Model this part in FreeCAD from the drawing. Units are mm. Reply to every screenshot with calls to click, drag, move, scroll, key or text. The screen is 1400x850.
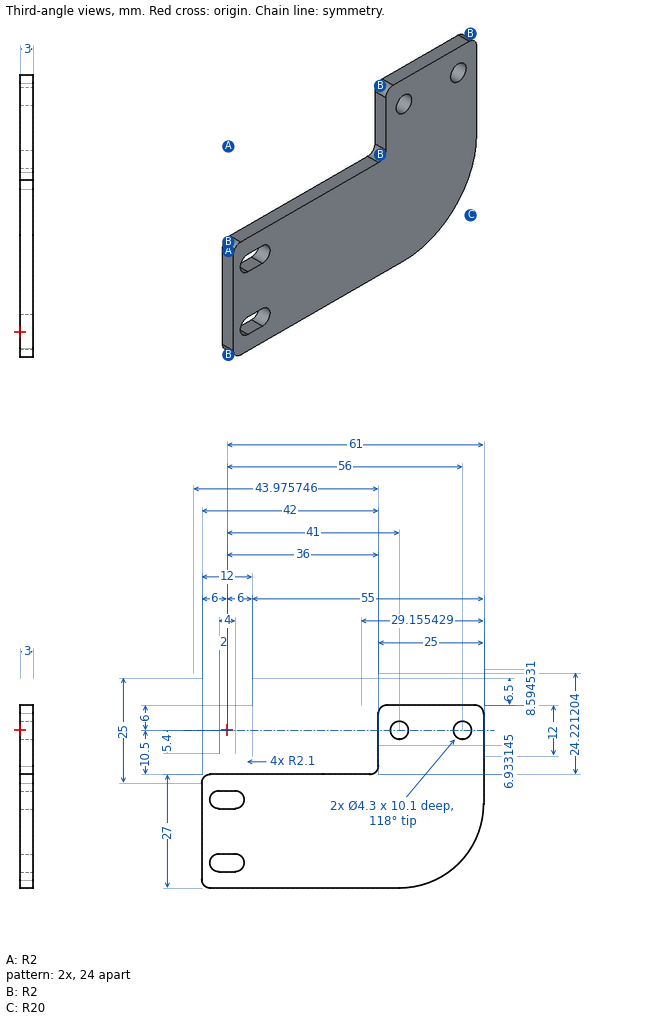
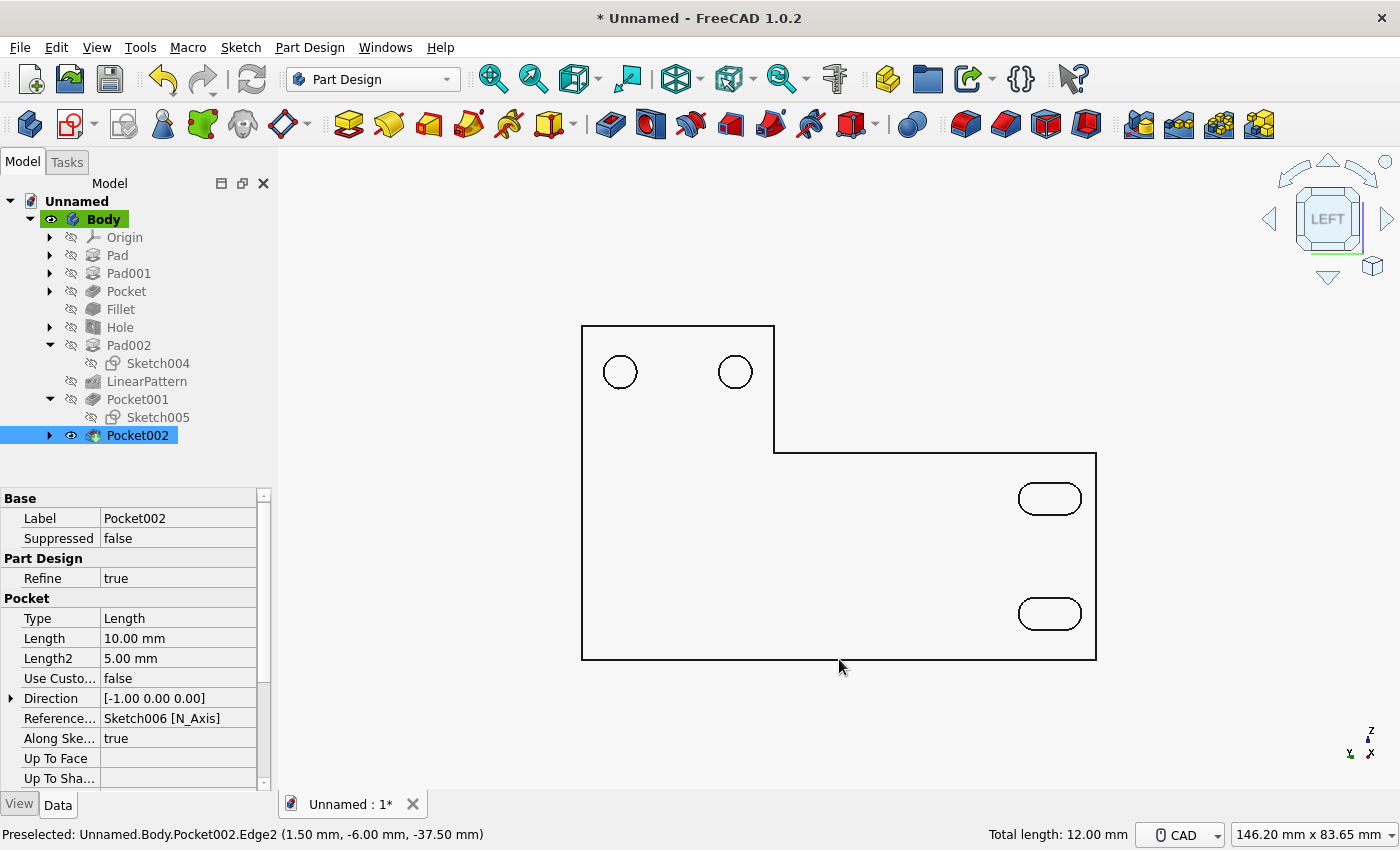
key(0)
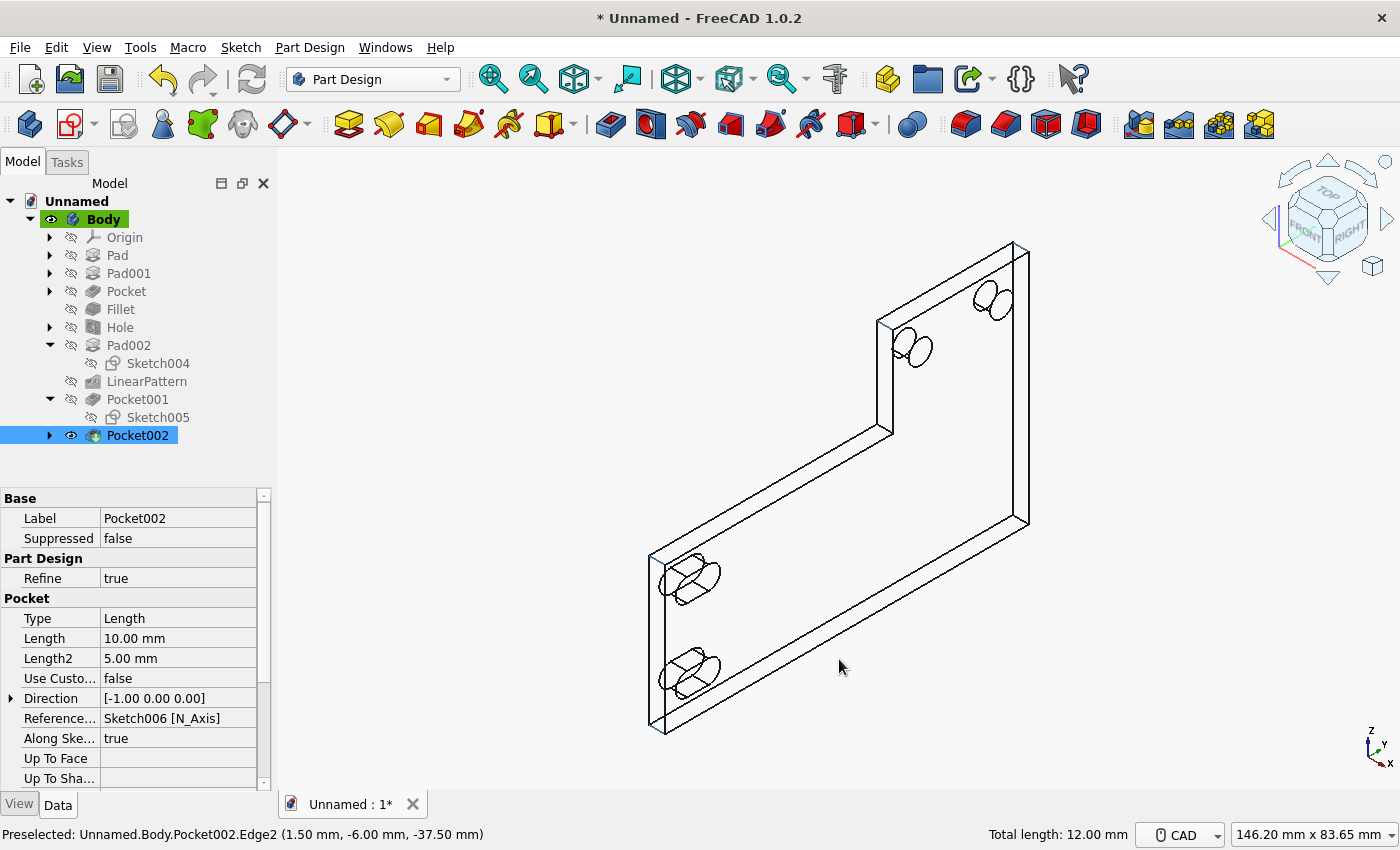
click(885, 428, ctrl)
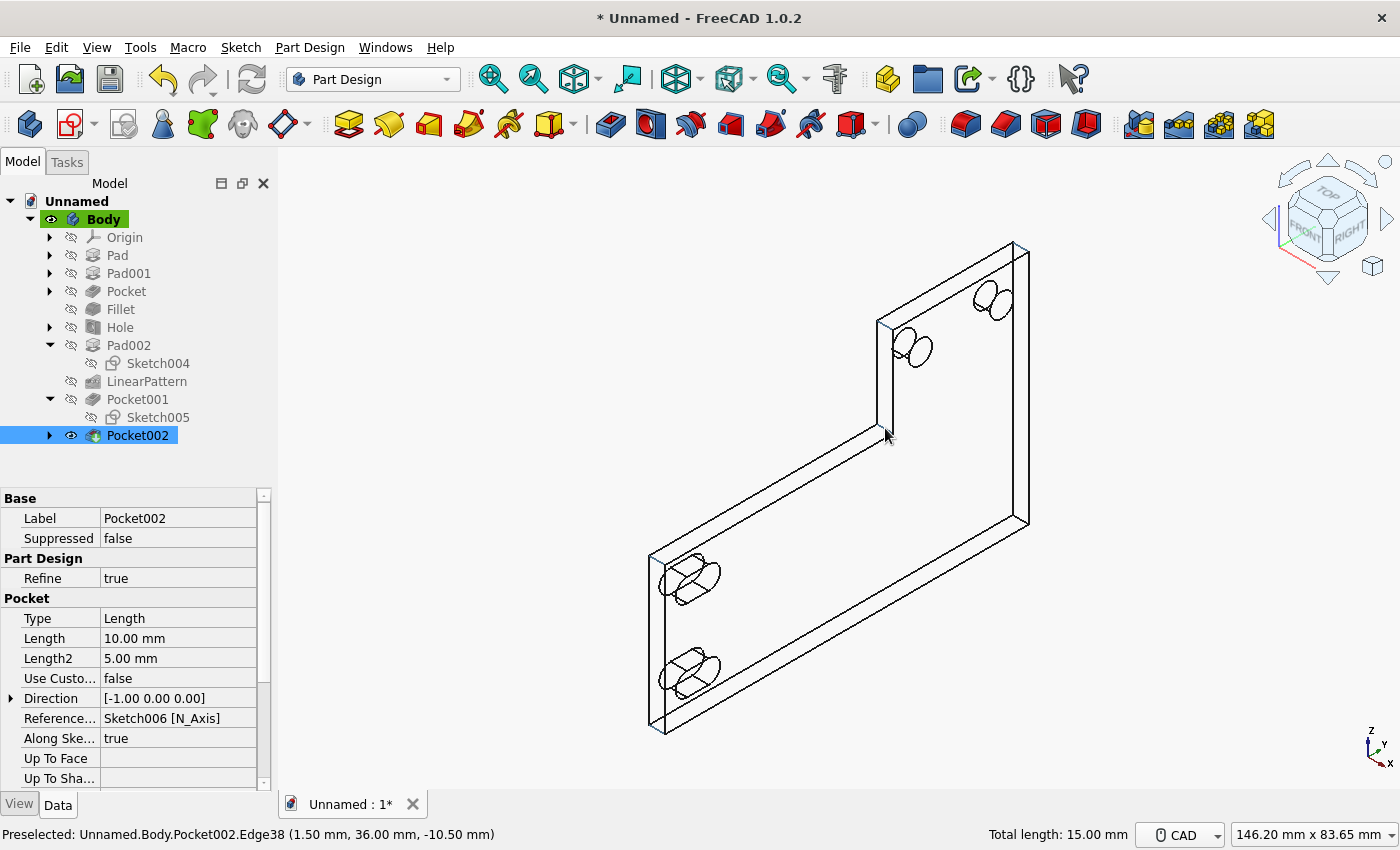
key(v)
key(1)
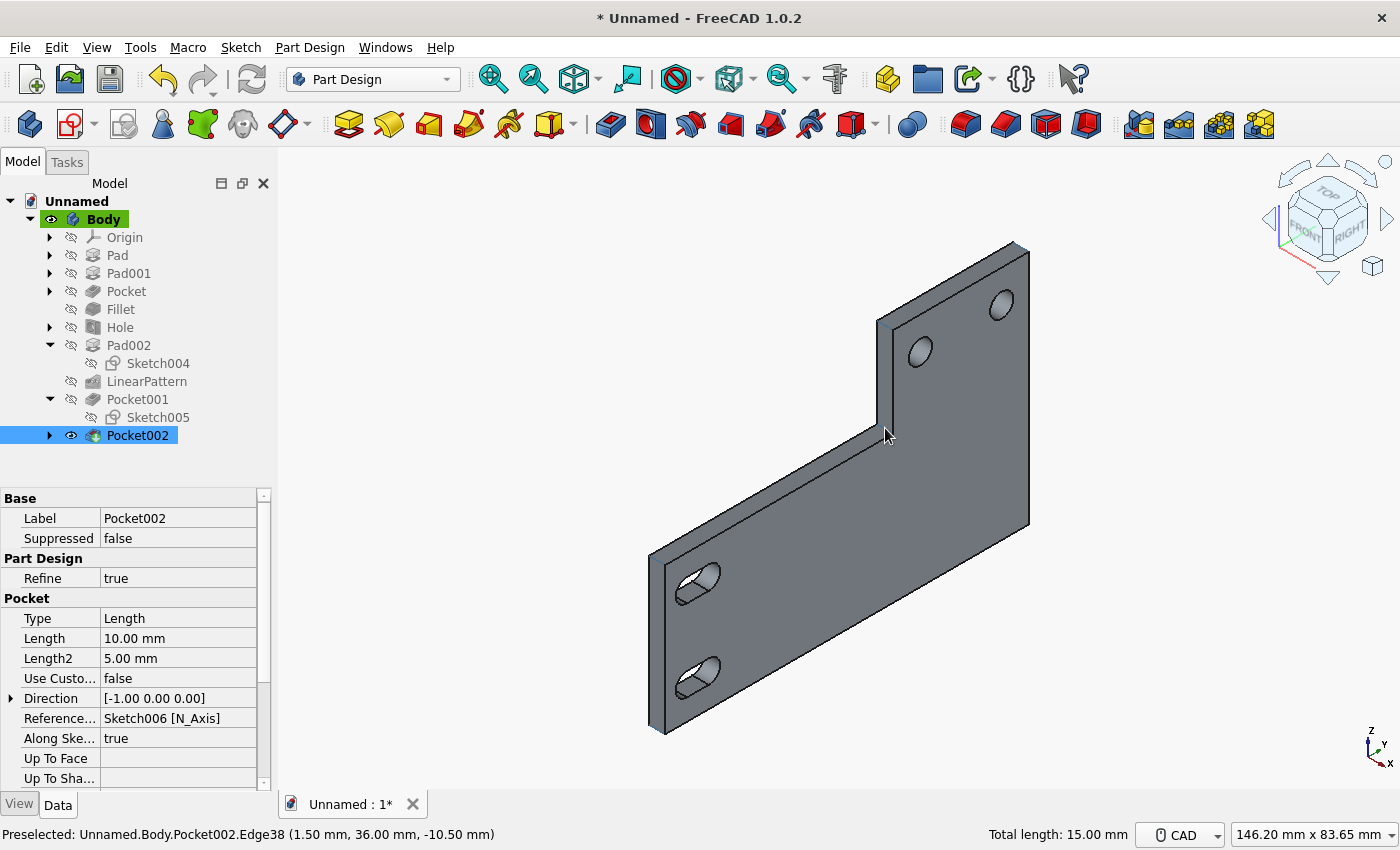
click(966, 124)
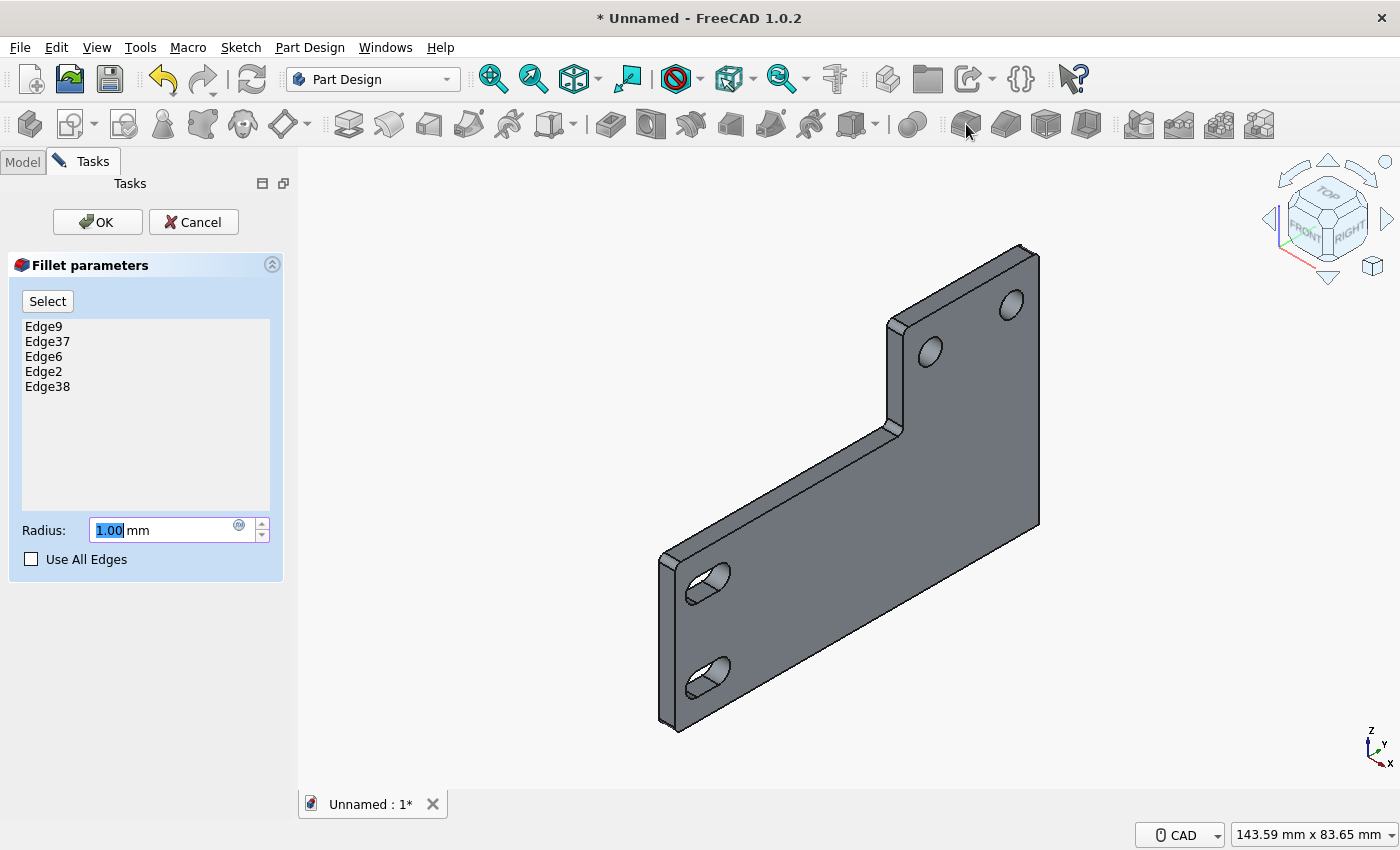
text(2)
key(Tab)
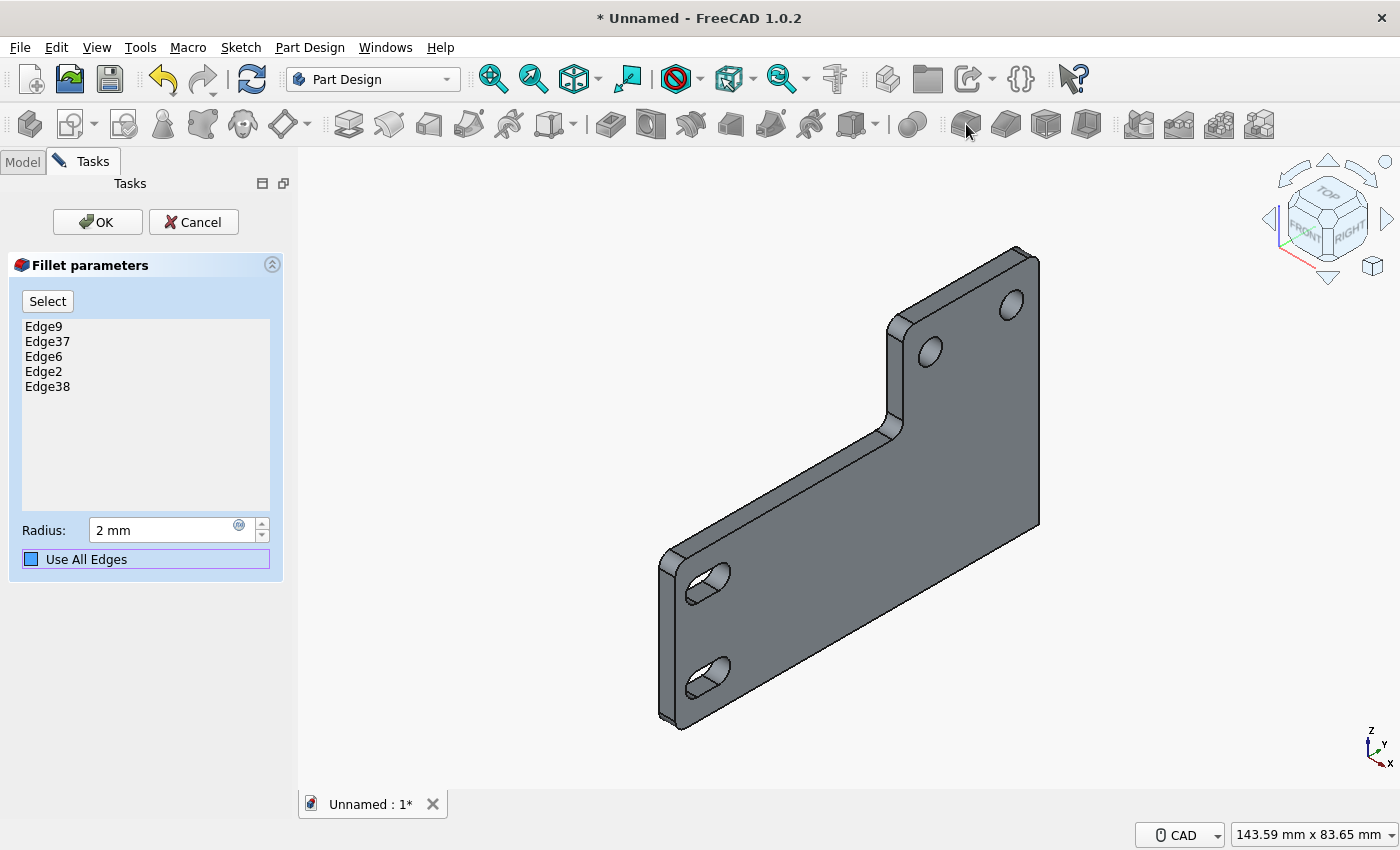
click(98, 222)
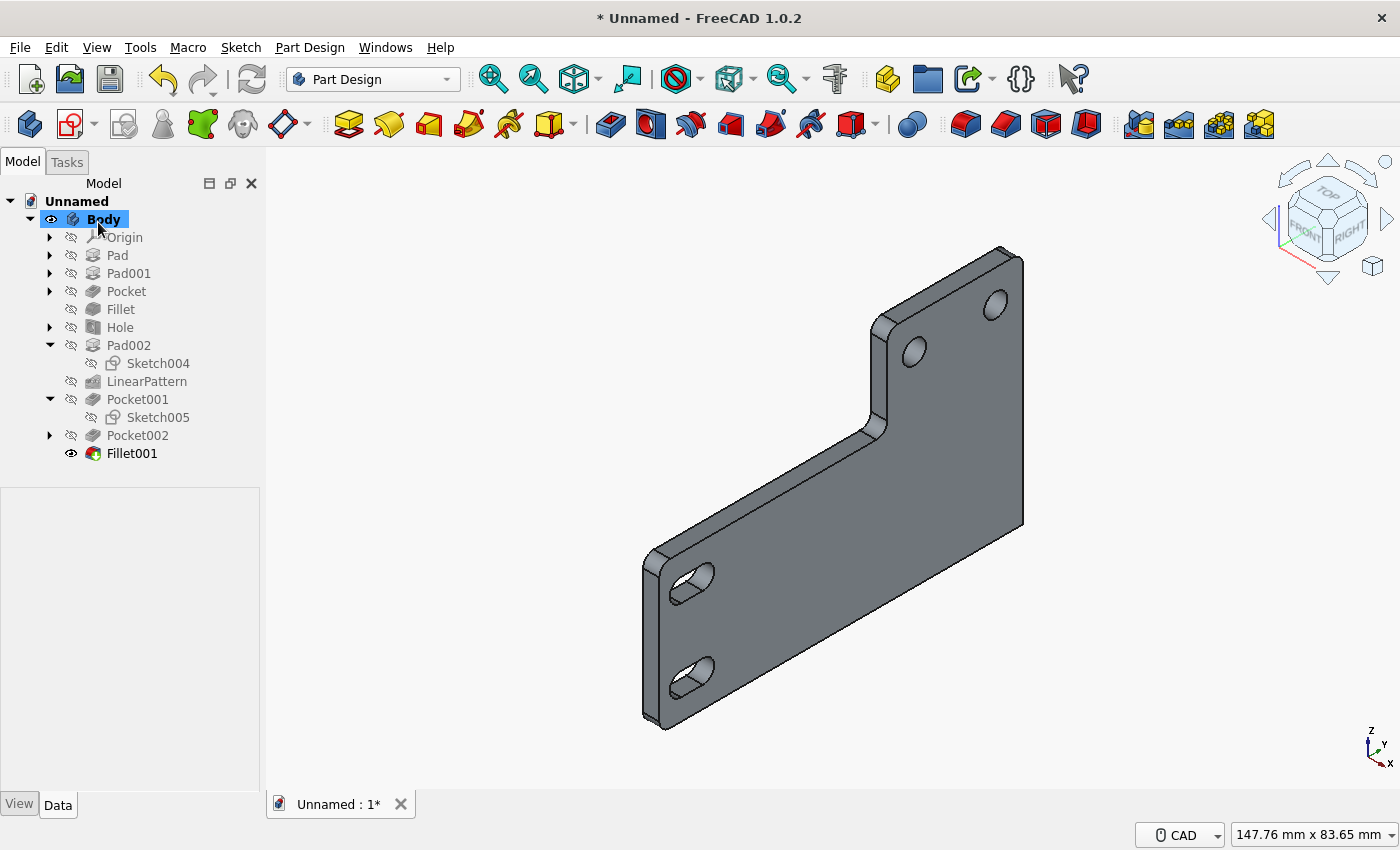
key(2)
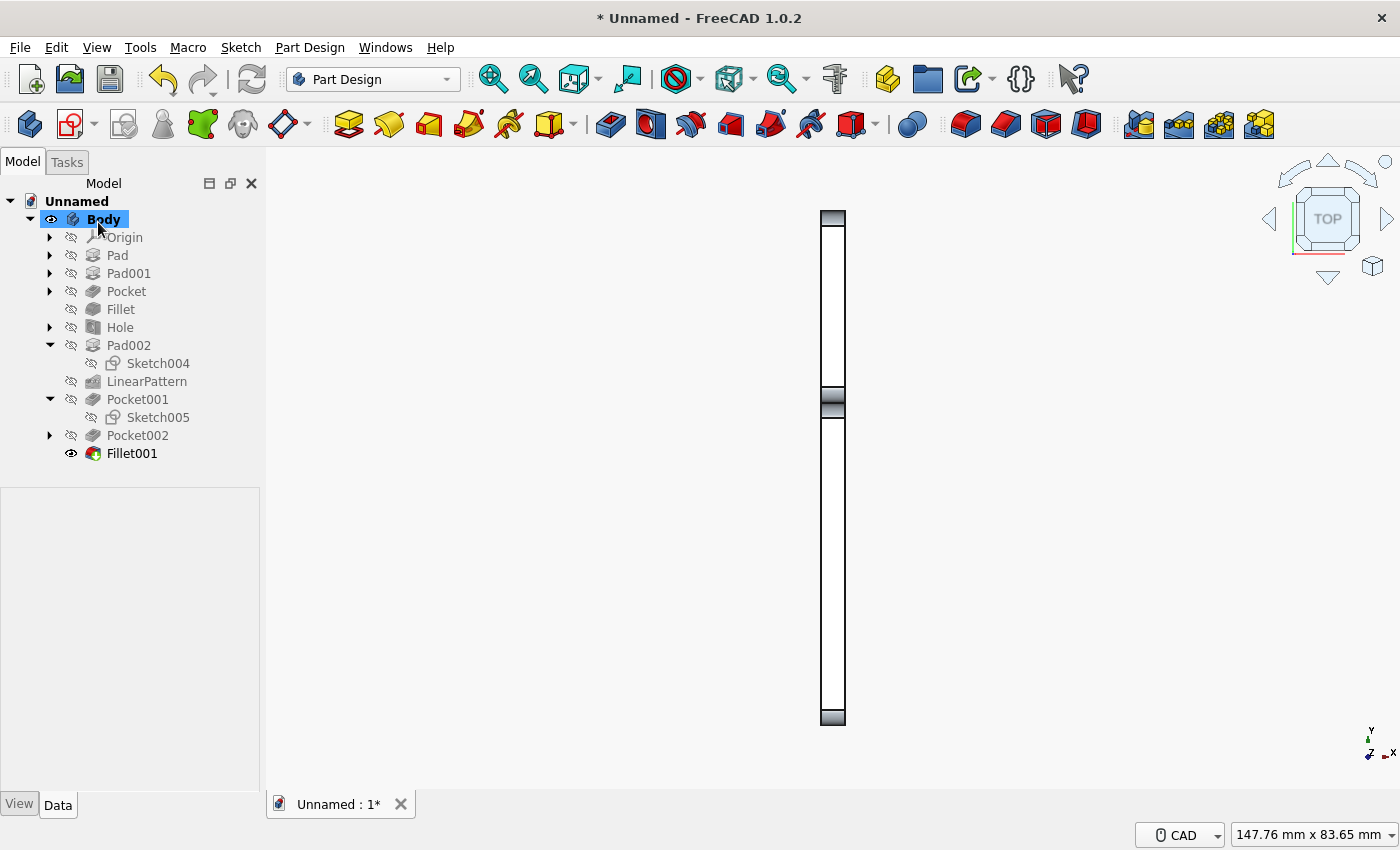
key(0)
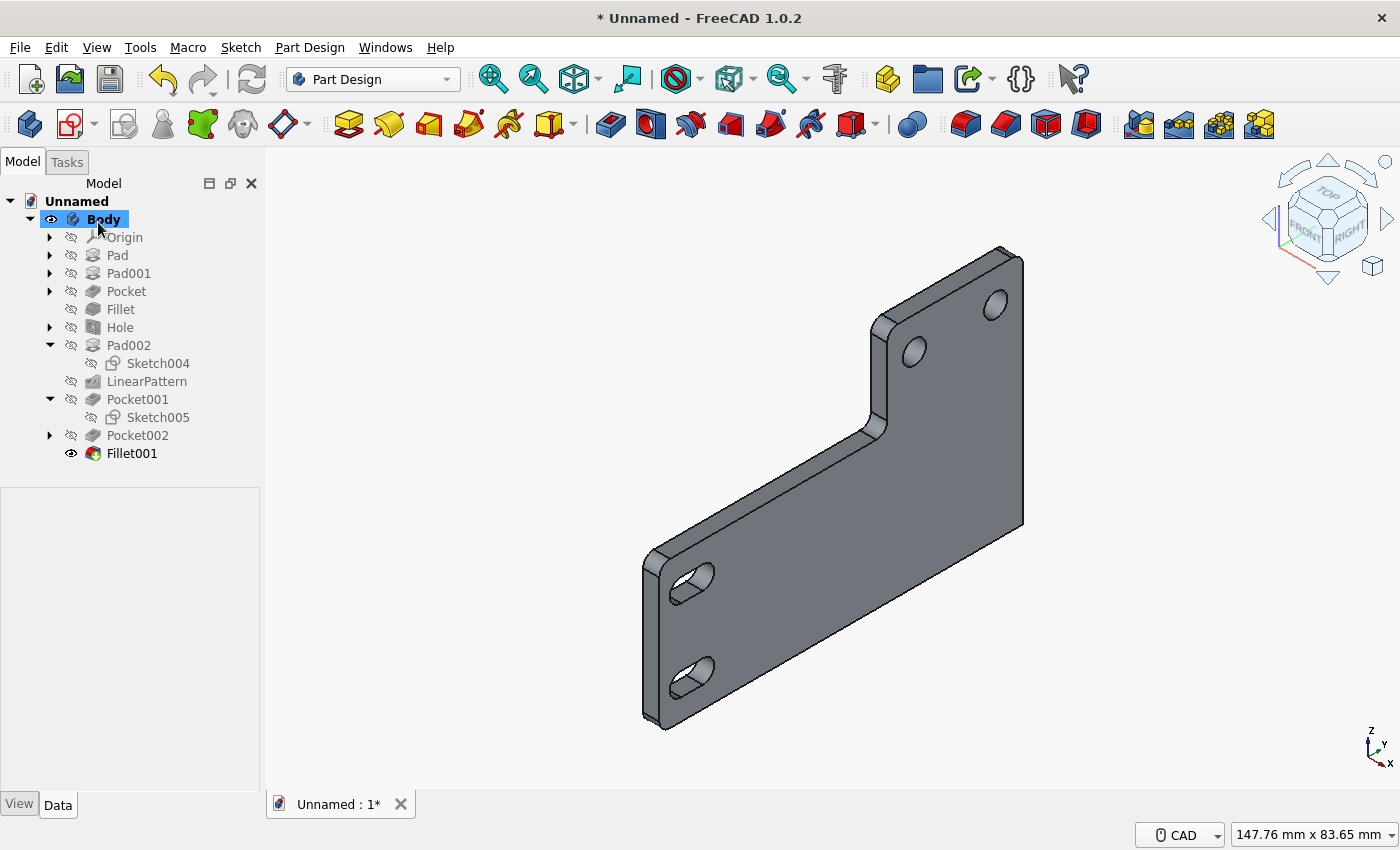
key(1)